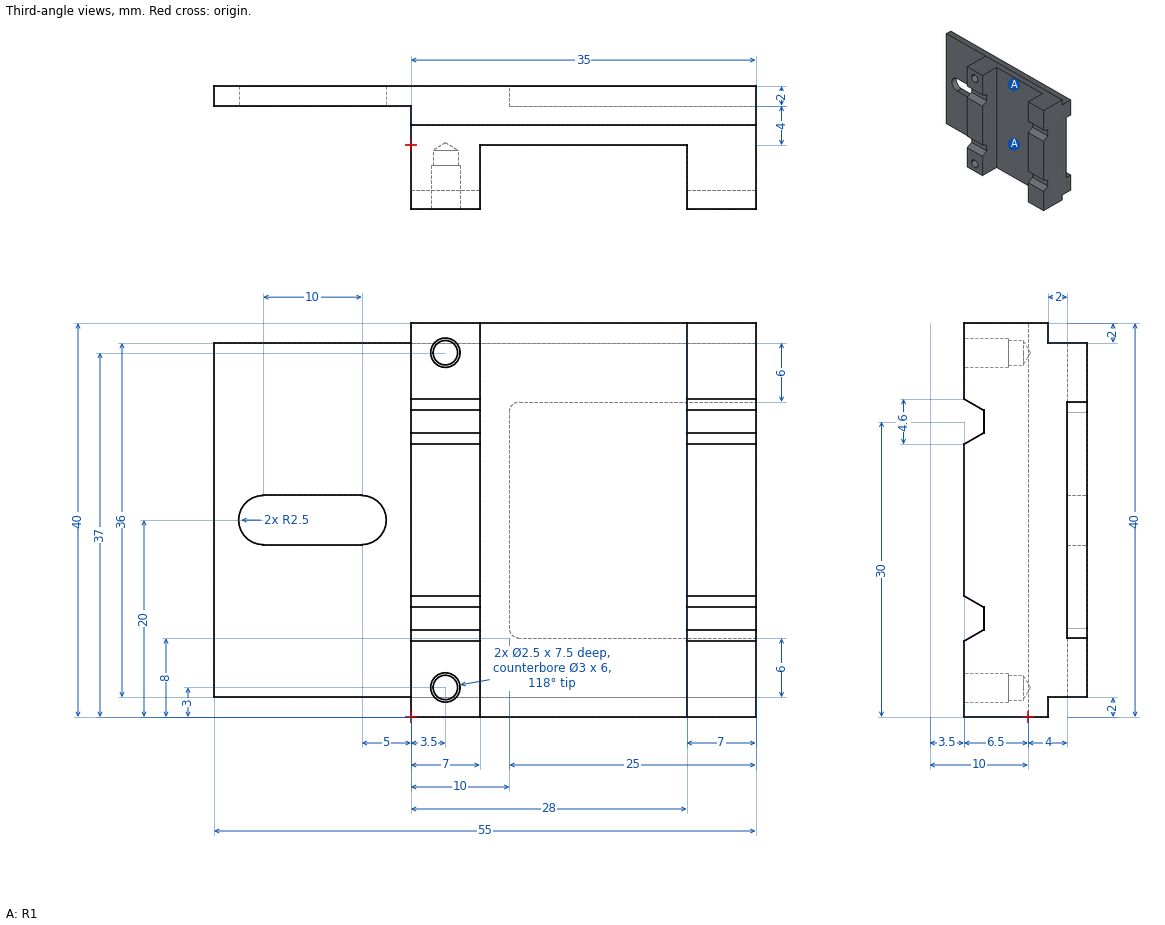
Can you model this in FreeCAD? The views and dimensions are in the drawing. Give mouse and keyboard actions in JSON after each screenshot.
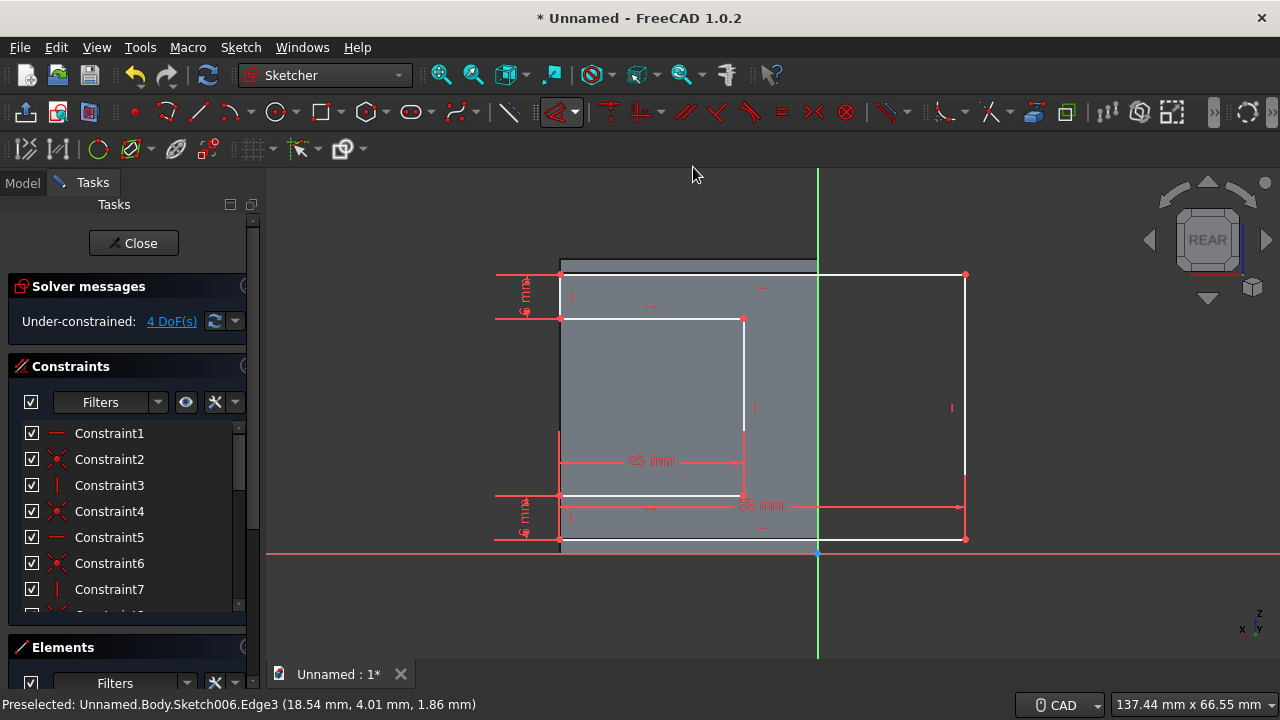
{"action": "left_click", "coordinate": [965, 460]}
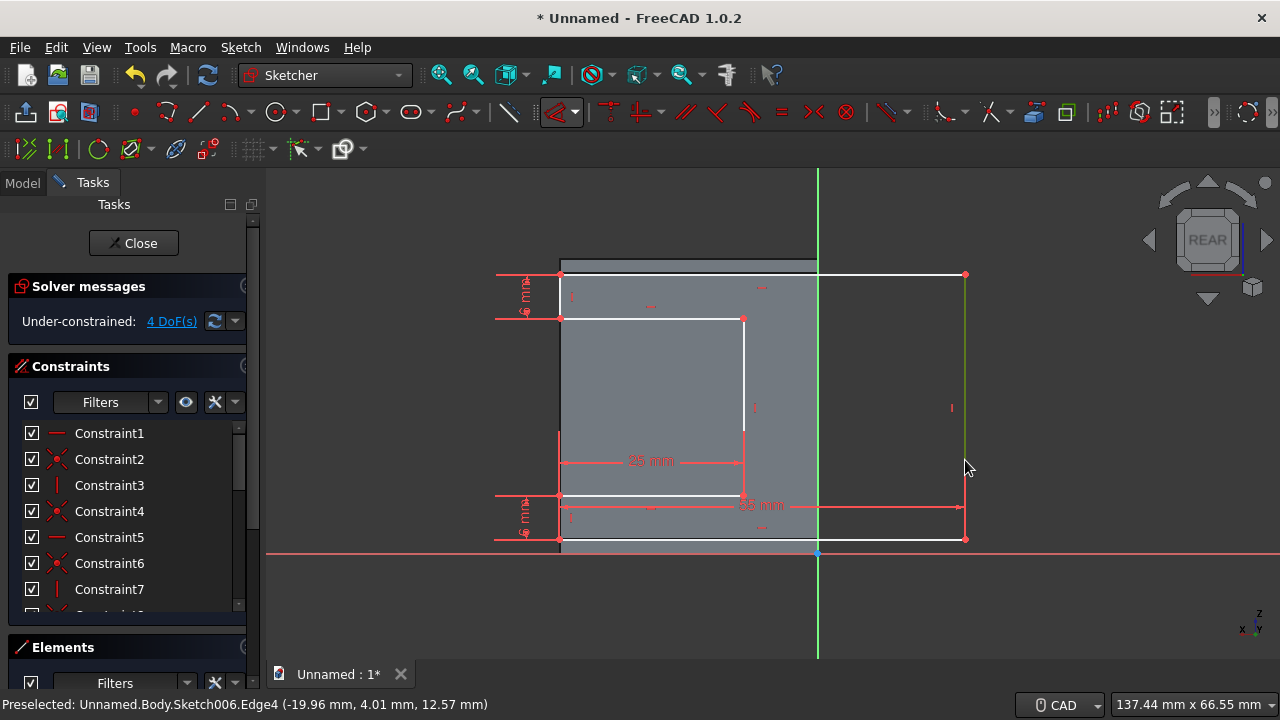
{"action": "key", "text": "i"}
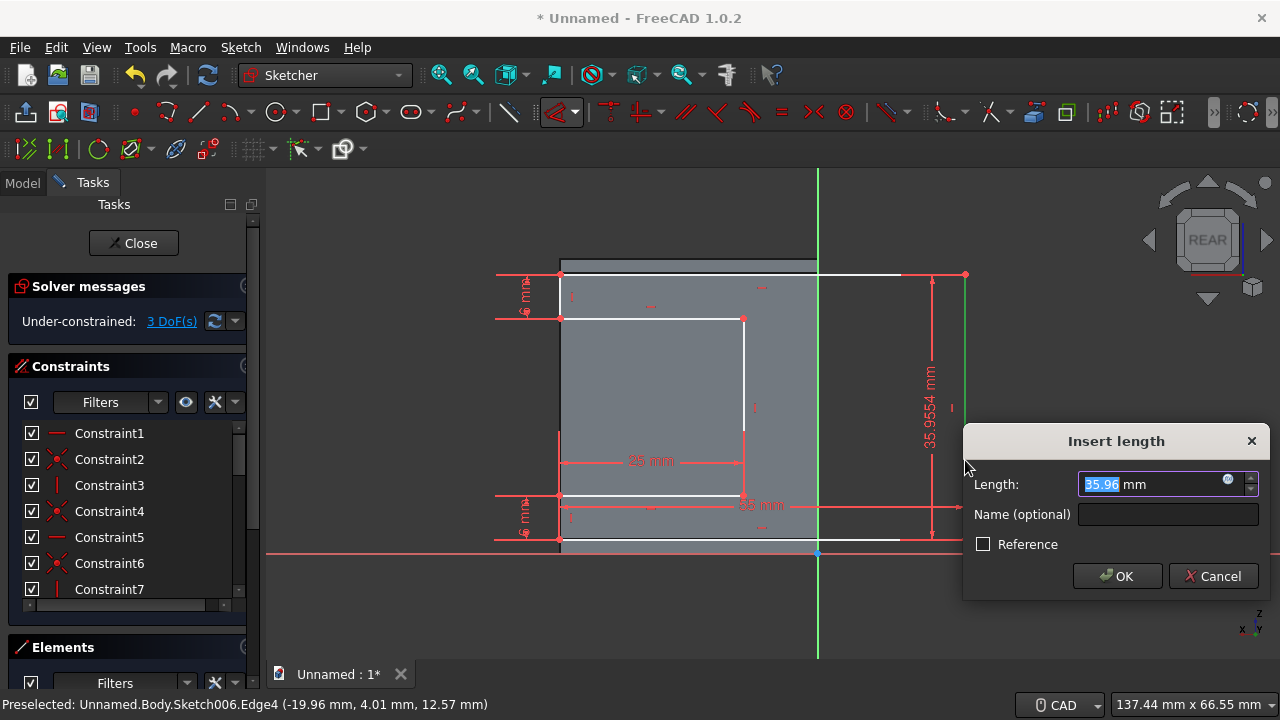
{"action": "type", "text": "36"}
{"action": "key", "text": "Return"}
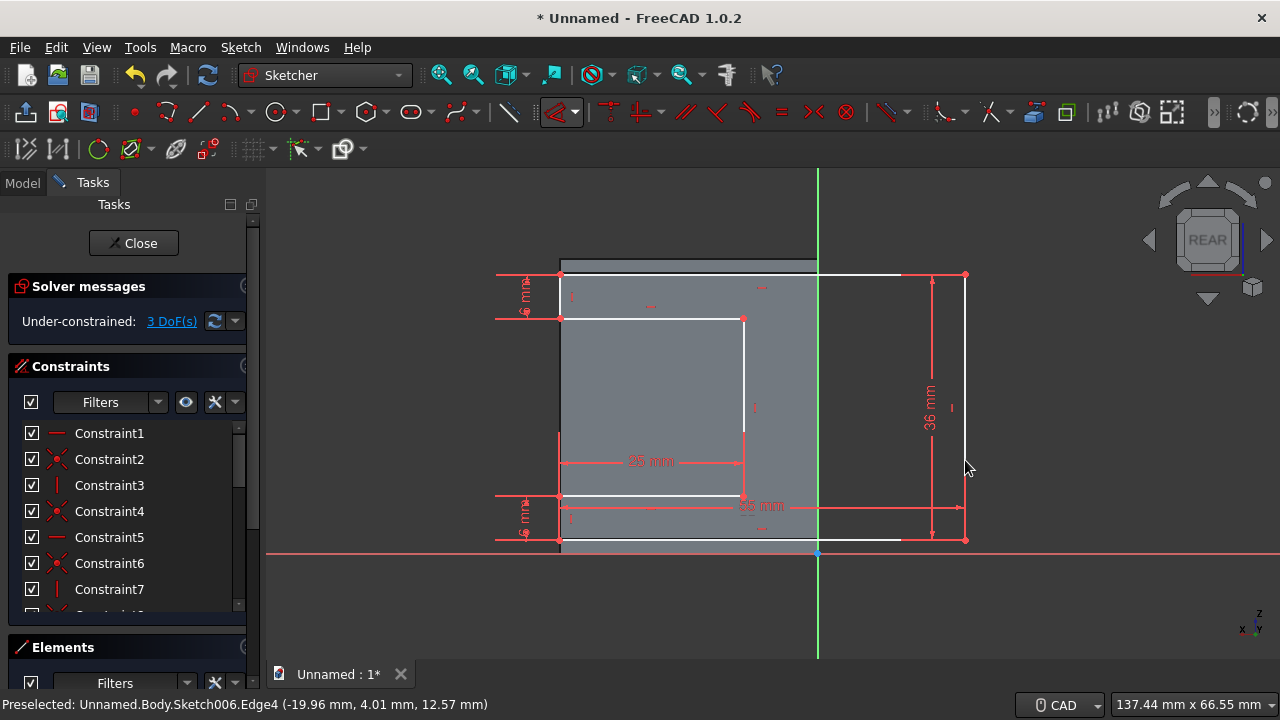
{"action": "left_click", "coordinate": [844, 275]}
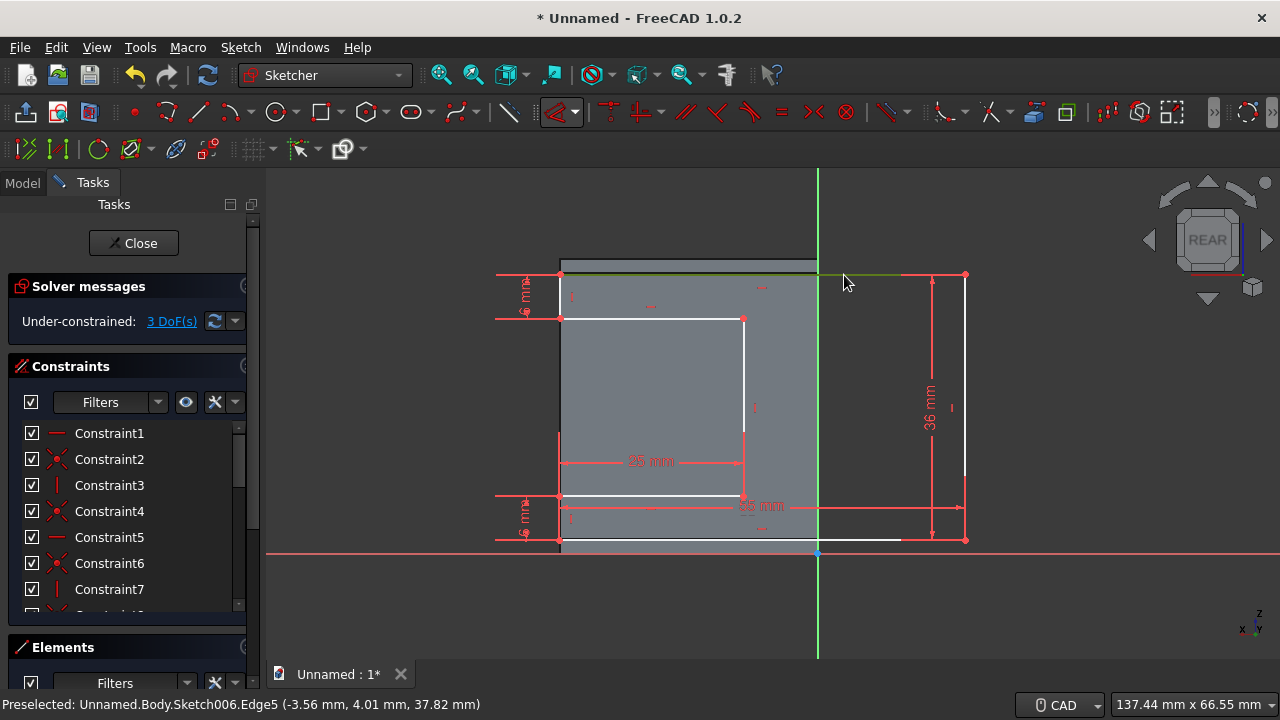
{"action": "key", "text": "l"}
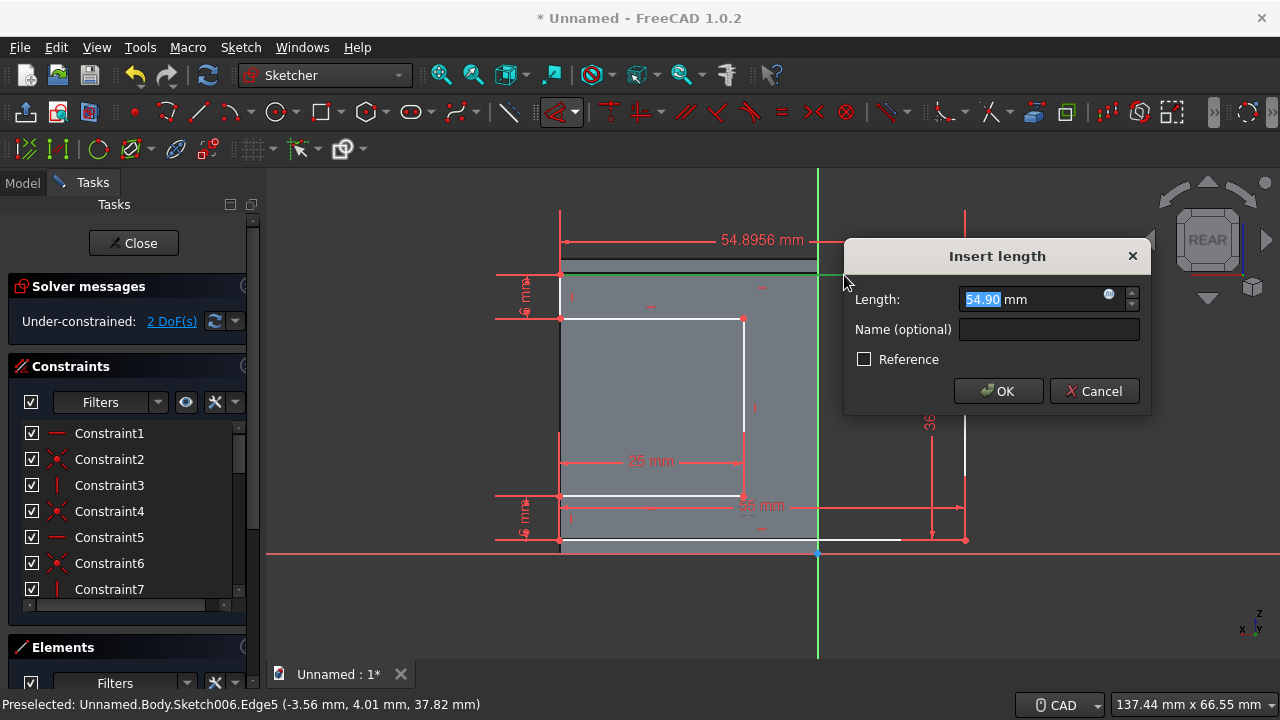
{"action": "type", "text": "55"}
{"action": "key", "text": "Return"}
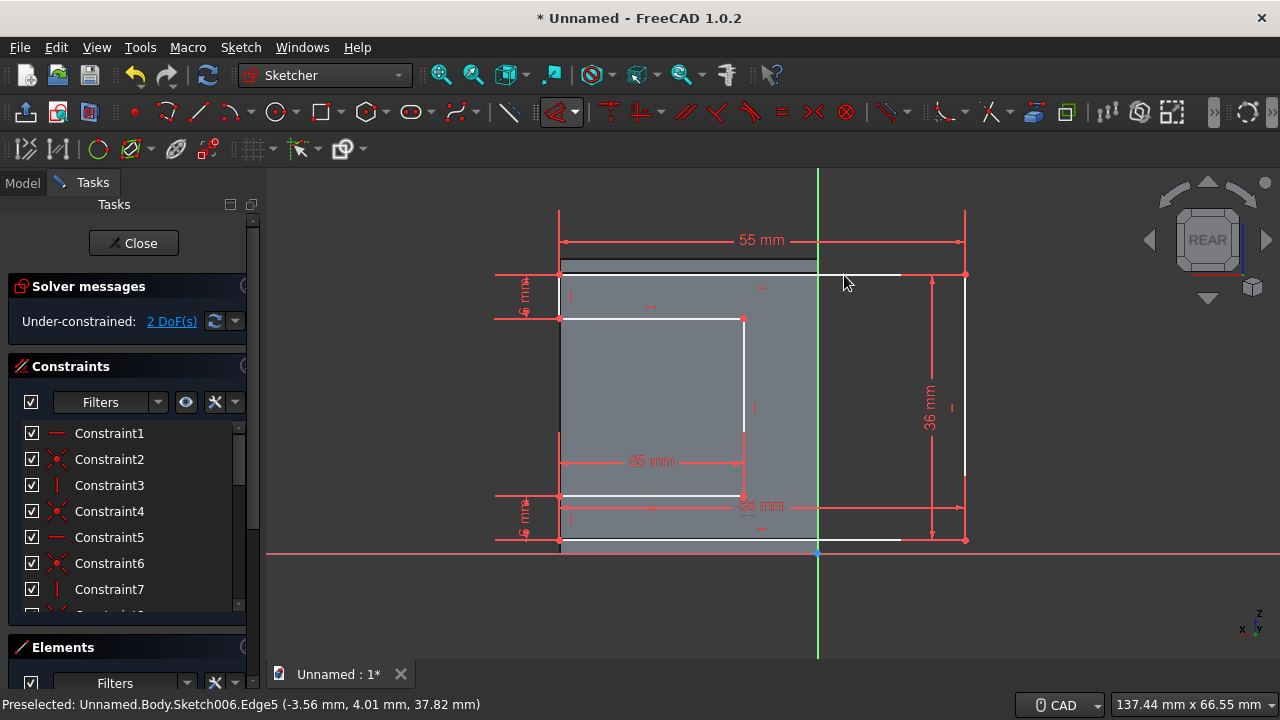
{"action": "left_click", "coordinate": [744, 496]}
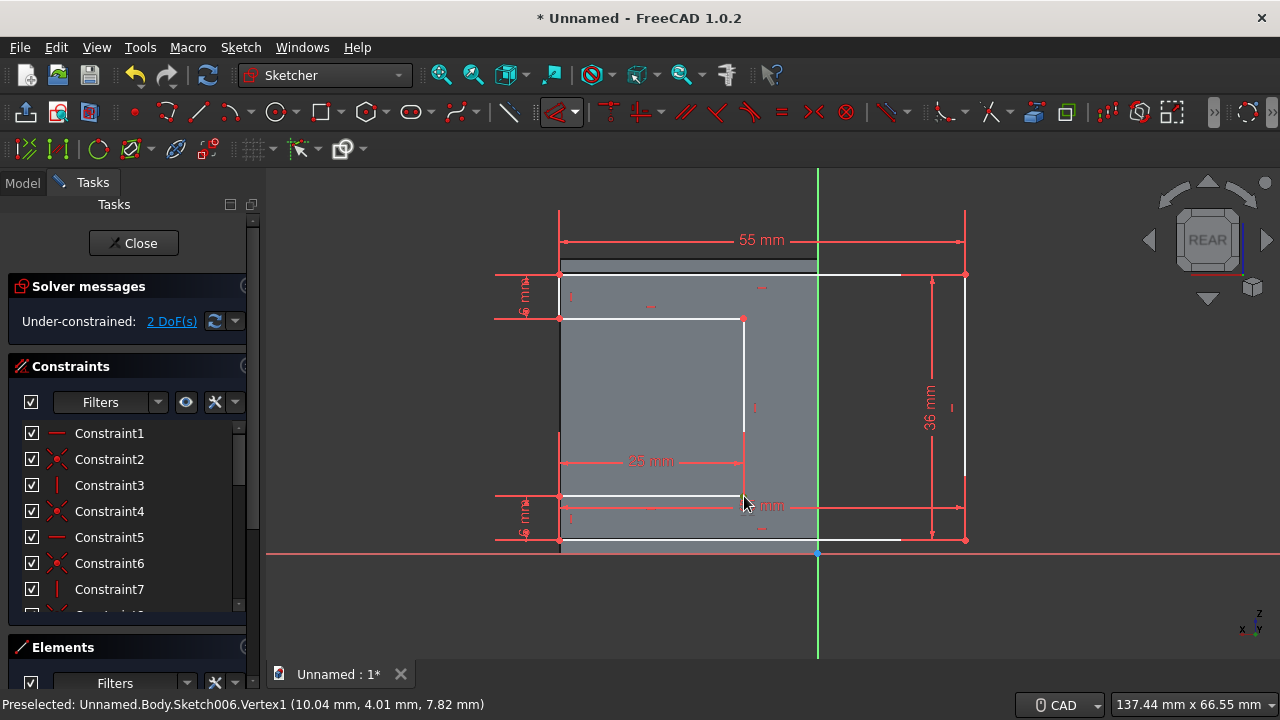
{"action": "key", "text": "i"}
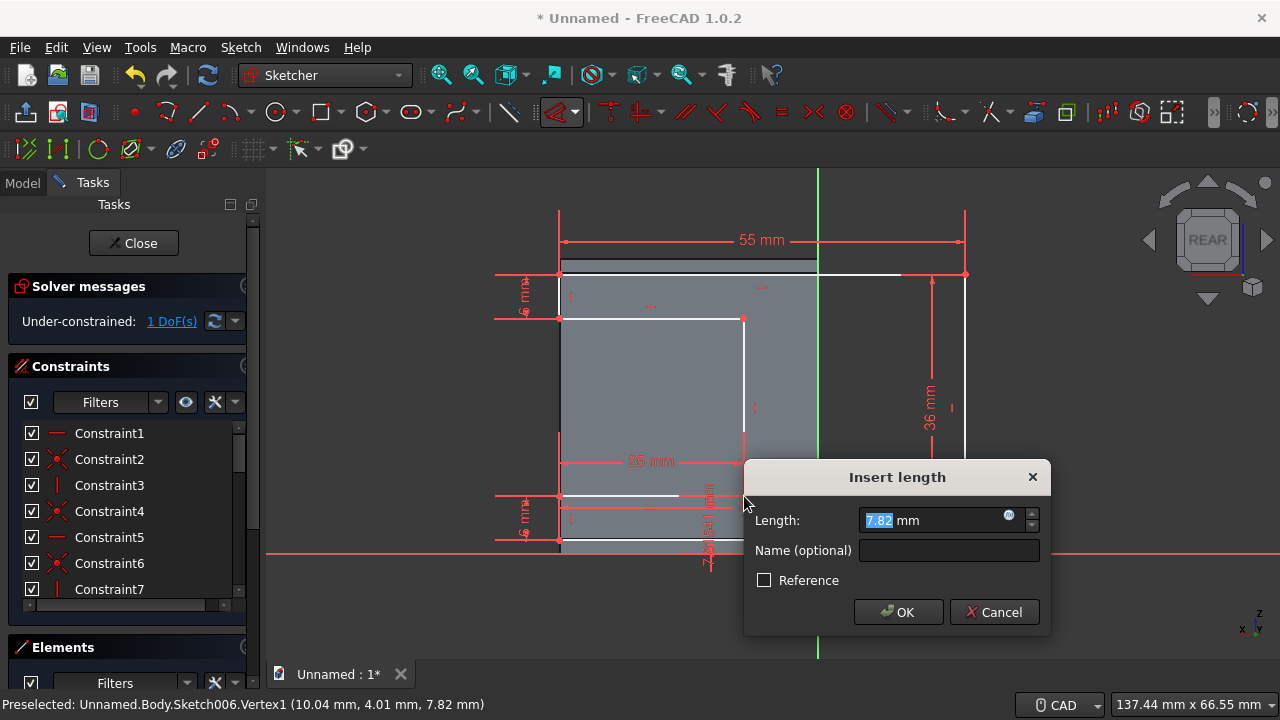
{"action": "type", "text": "8"}
{"action": "key", "text": "Return"}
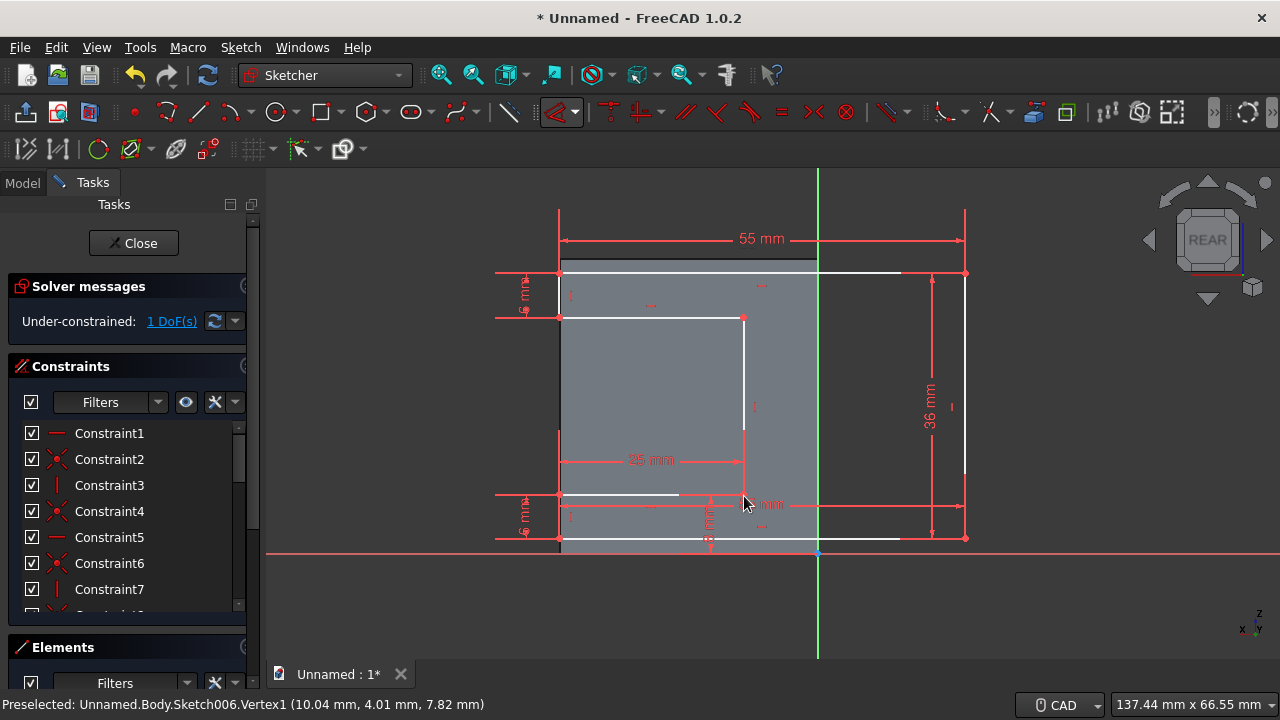
{"action": "left_click", "coordinate": [744, 495]}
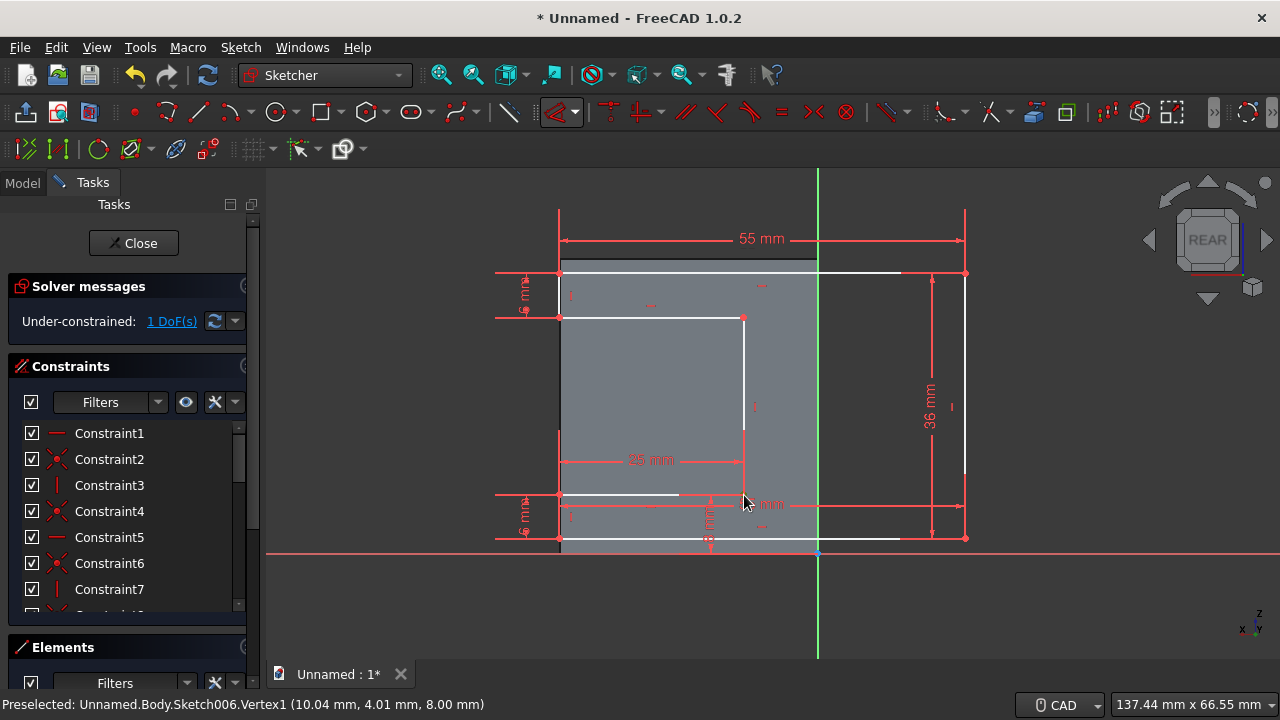
{"action": "left_click", "coordinate": [578, 112]}